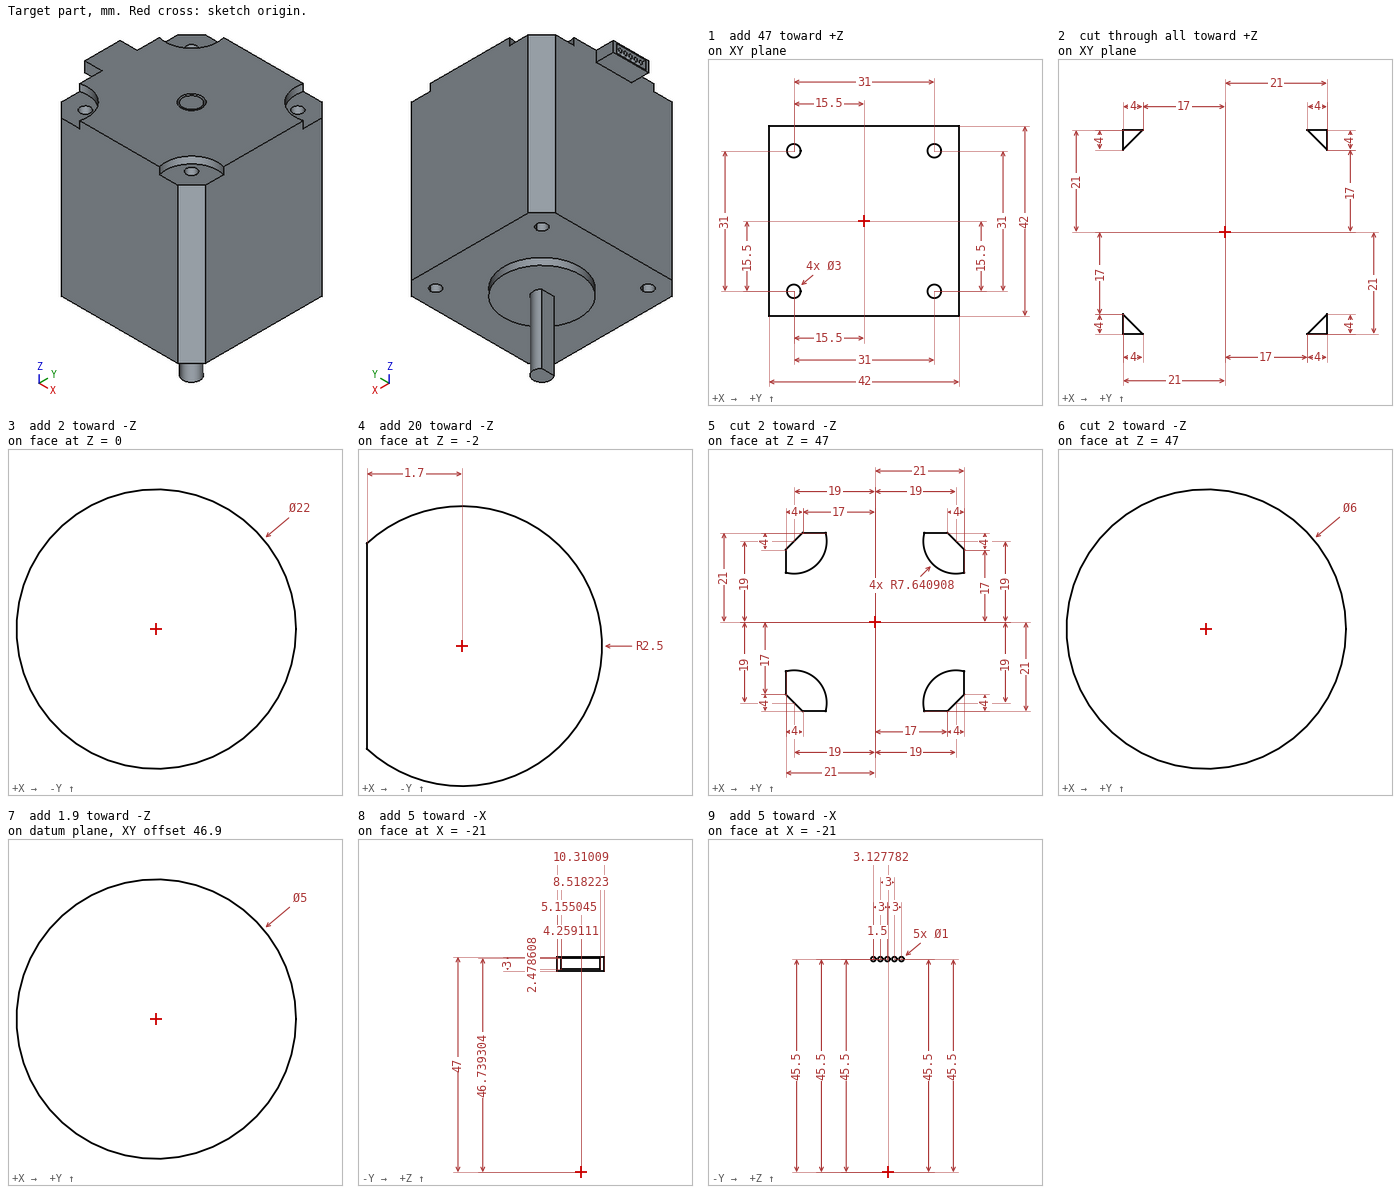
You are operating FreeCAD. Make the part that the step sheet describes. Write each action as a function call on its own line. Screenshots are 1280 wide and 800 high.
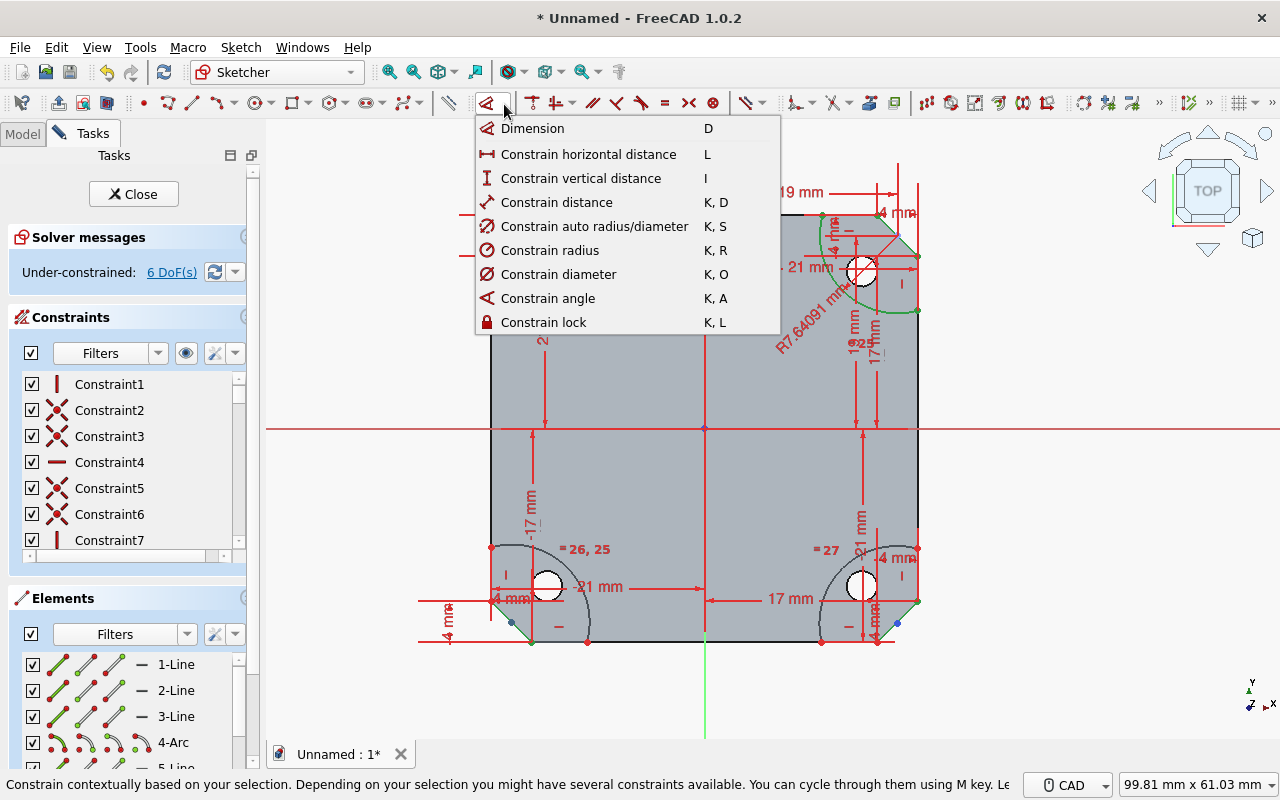
click(628, 154)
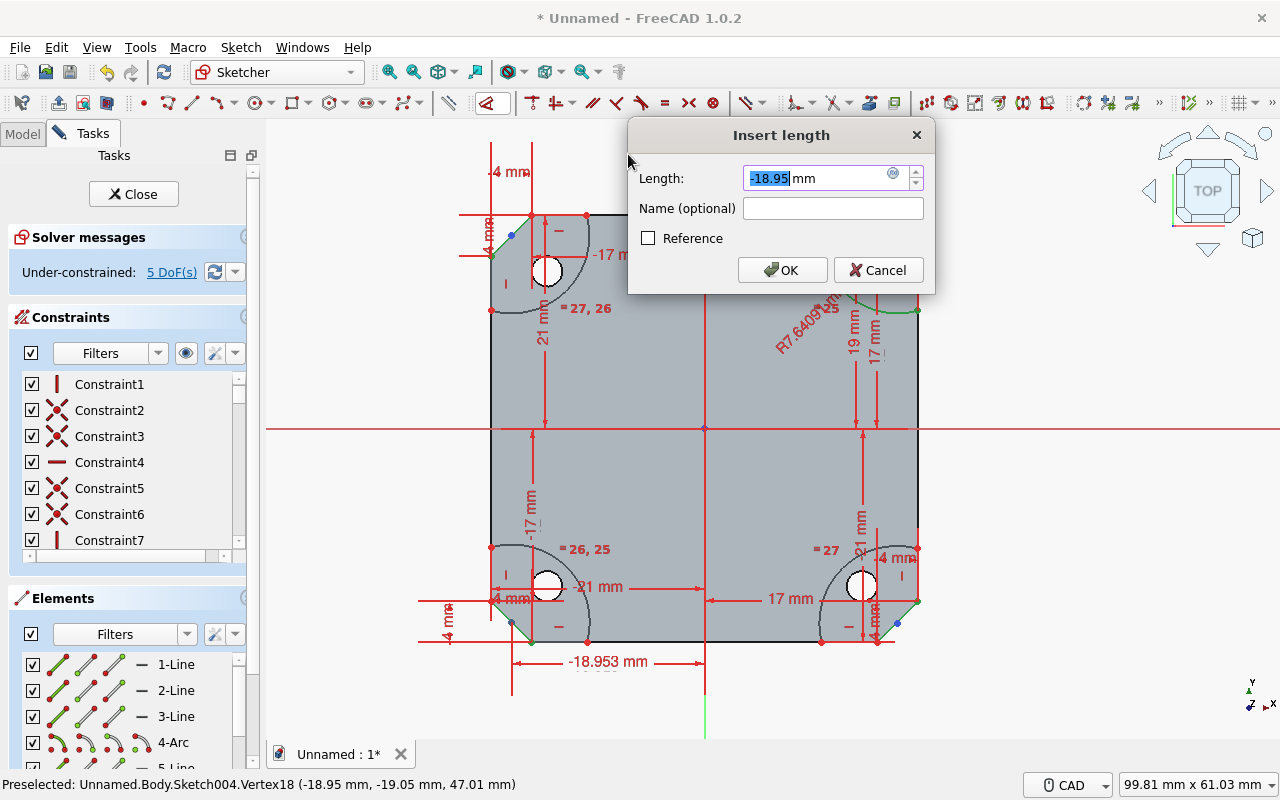
text(-19)
key(Return)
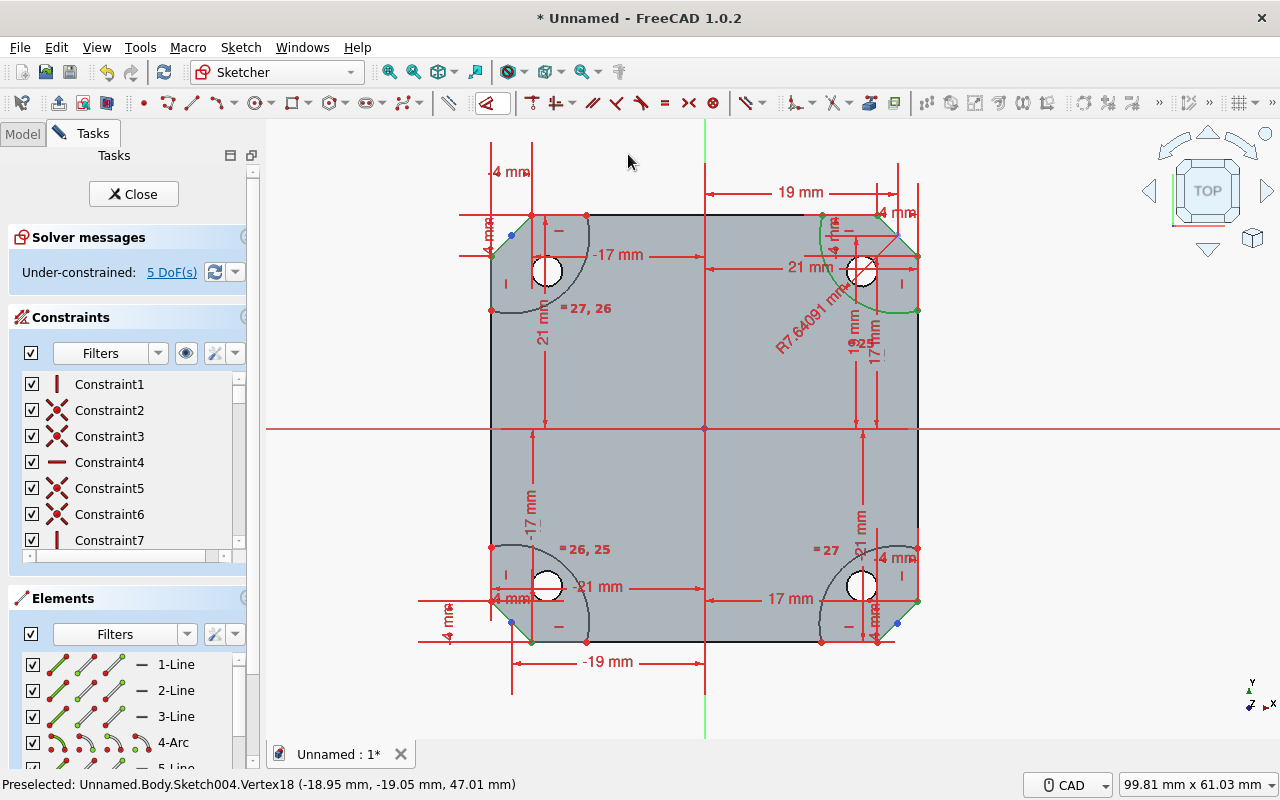
click(512, 622)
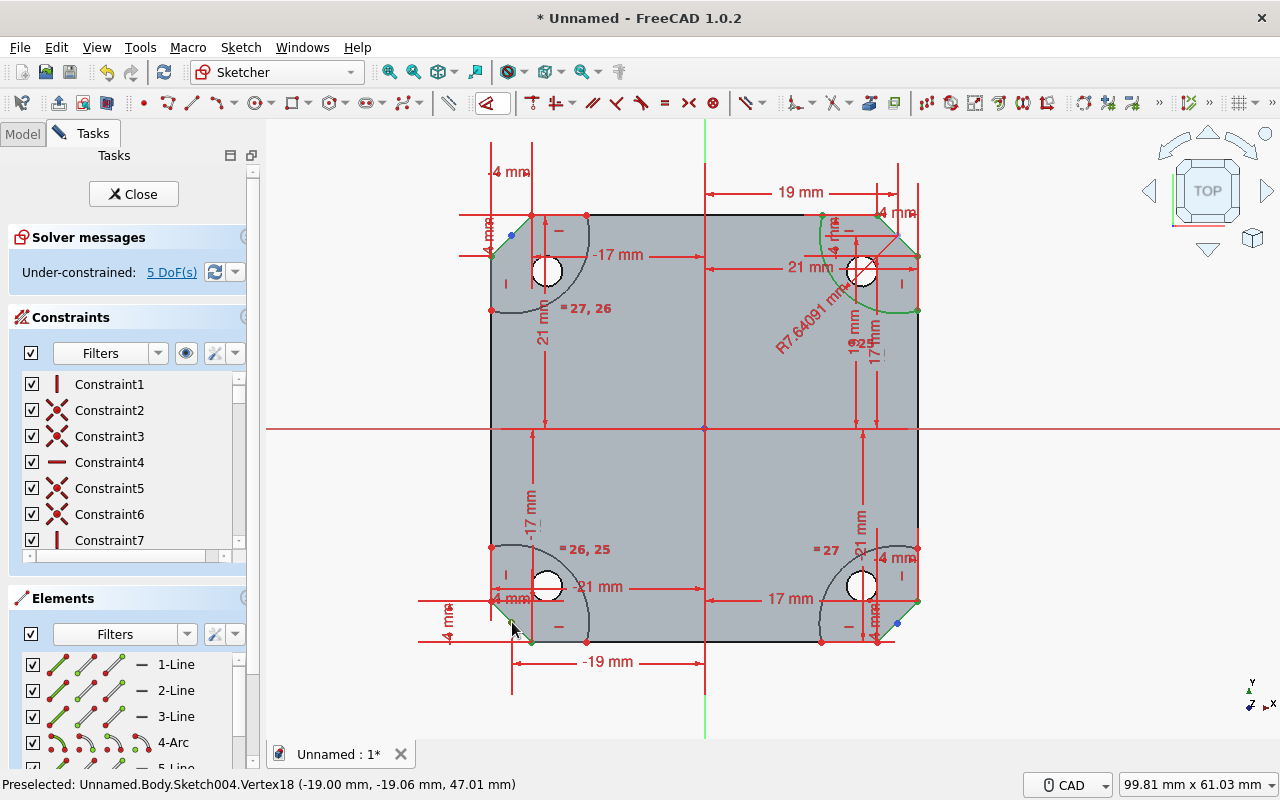
click(504, 104)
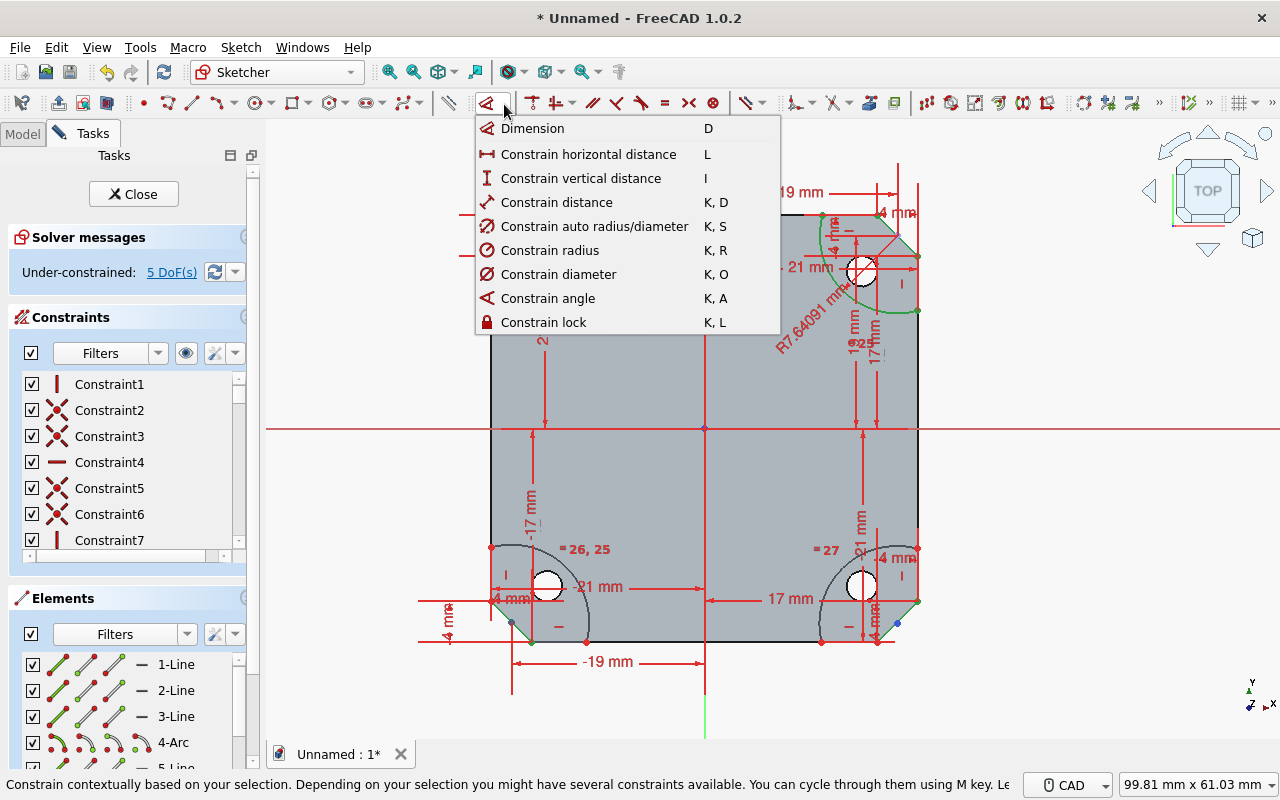
click(628, 178)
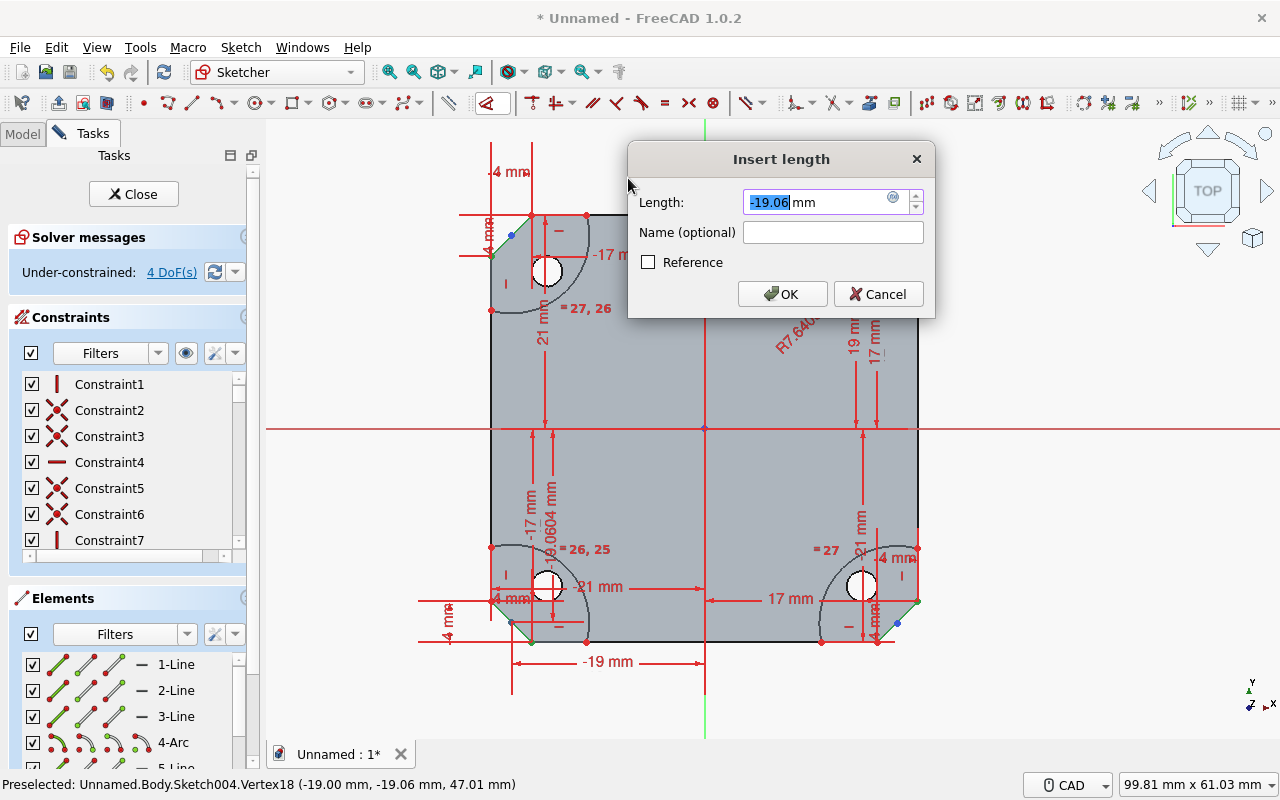
text(-19)
key(Return)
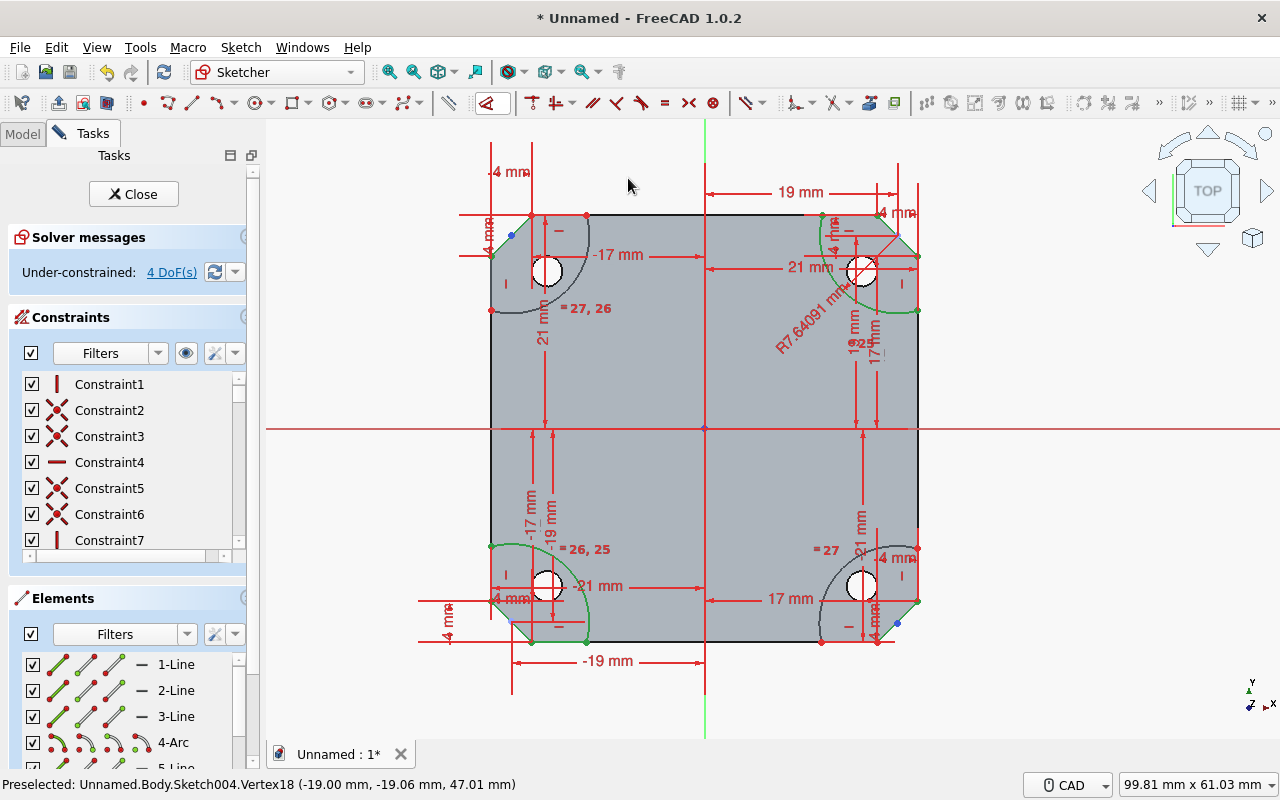
click(512, 236)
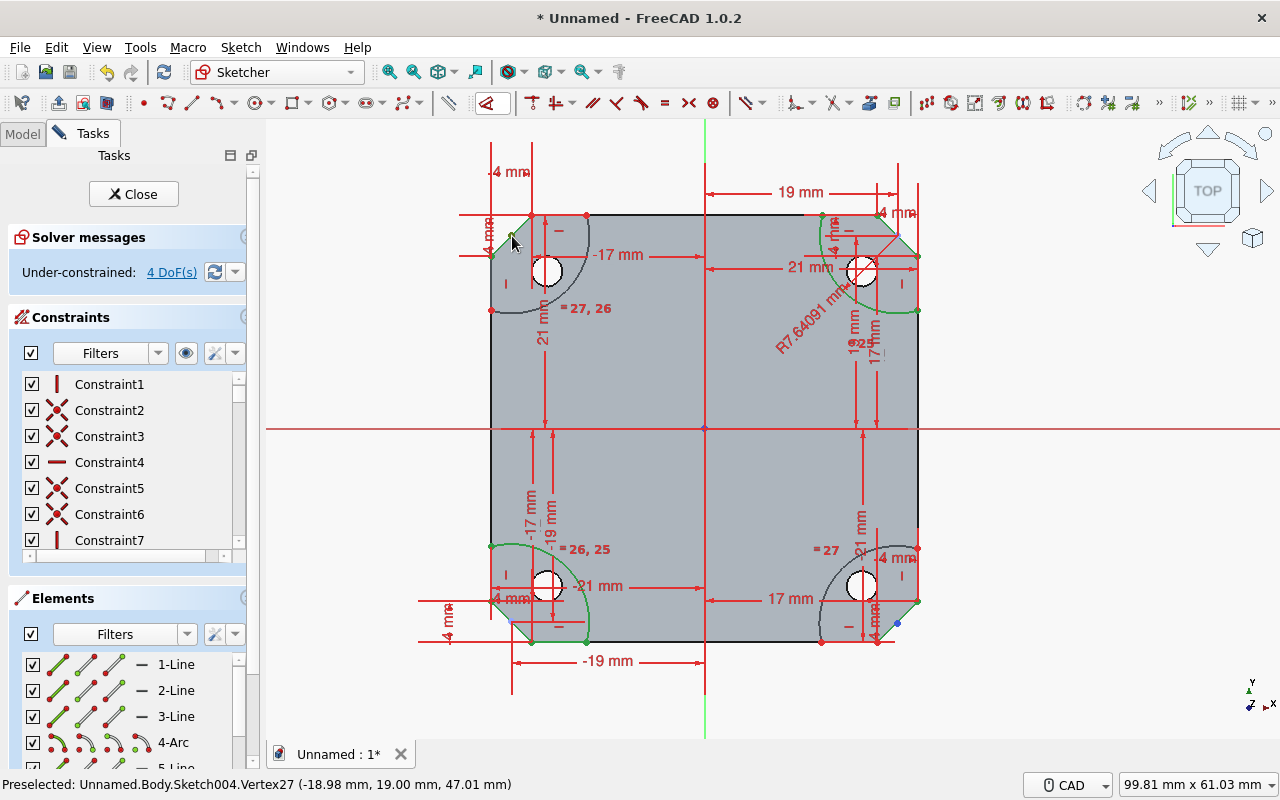
key(l)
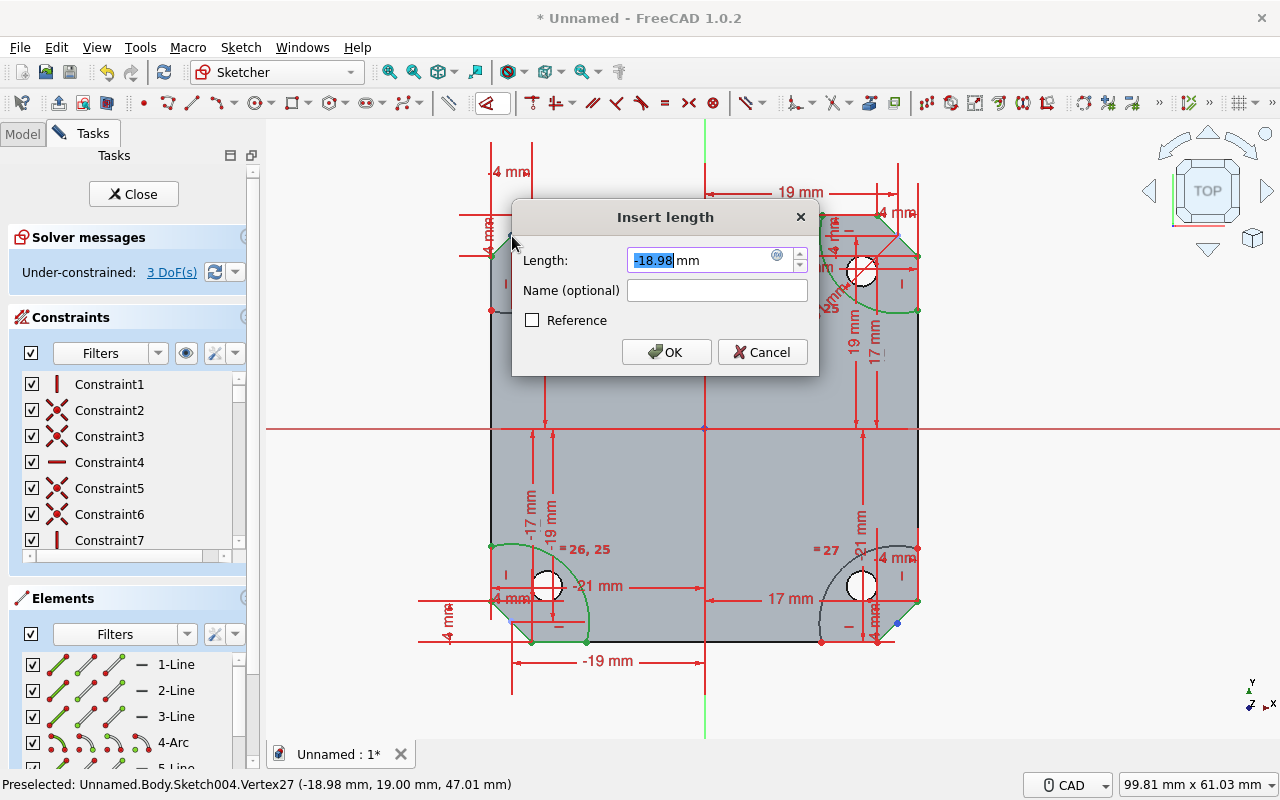
text(-19)
key(Return)